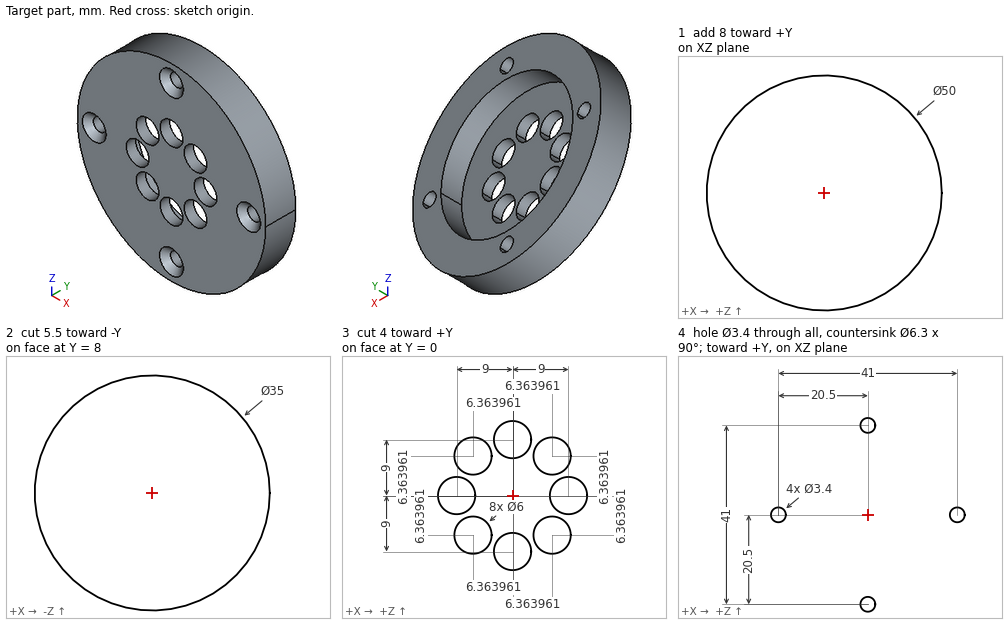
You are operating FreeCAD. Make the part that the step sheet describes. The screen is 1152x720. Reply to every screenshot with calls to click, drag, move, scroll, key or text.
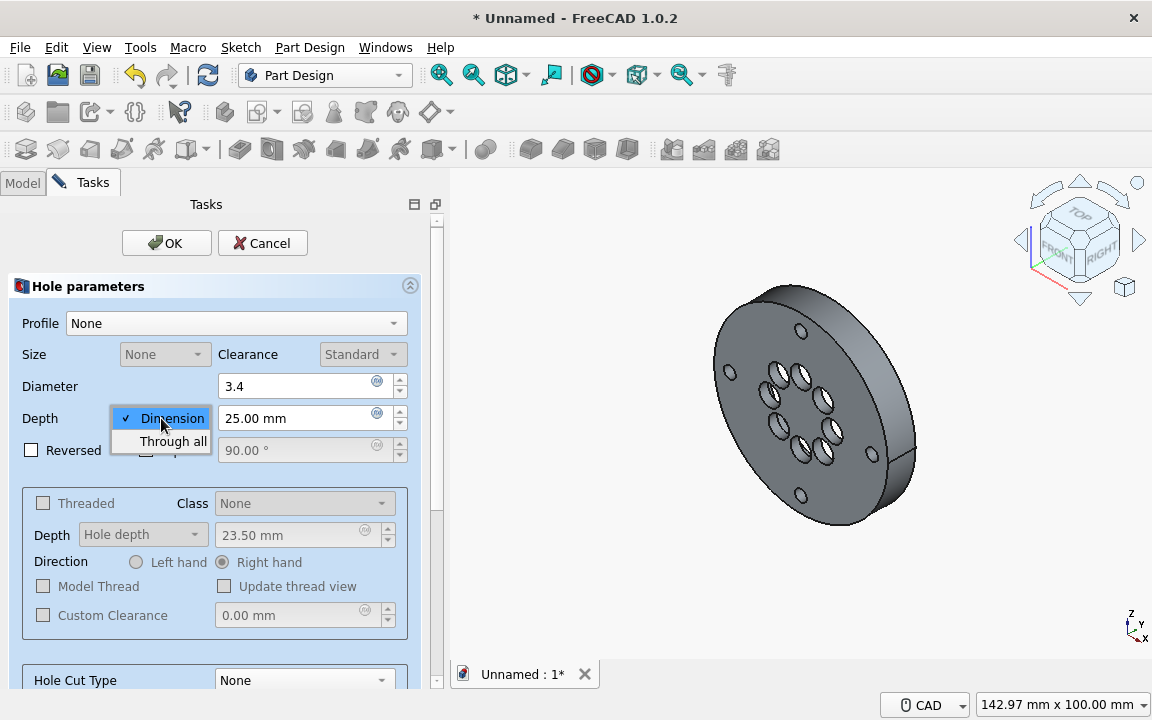
click(160, 442)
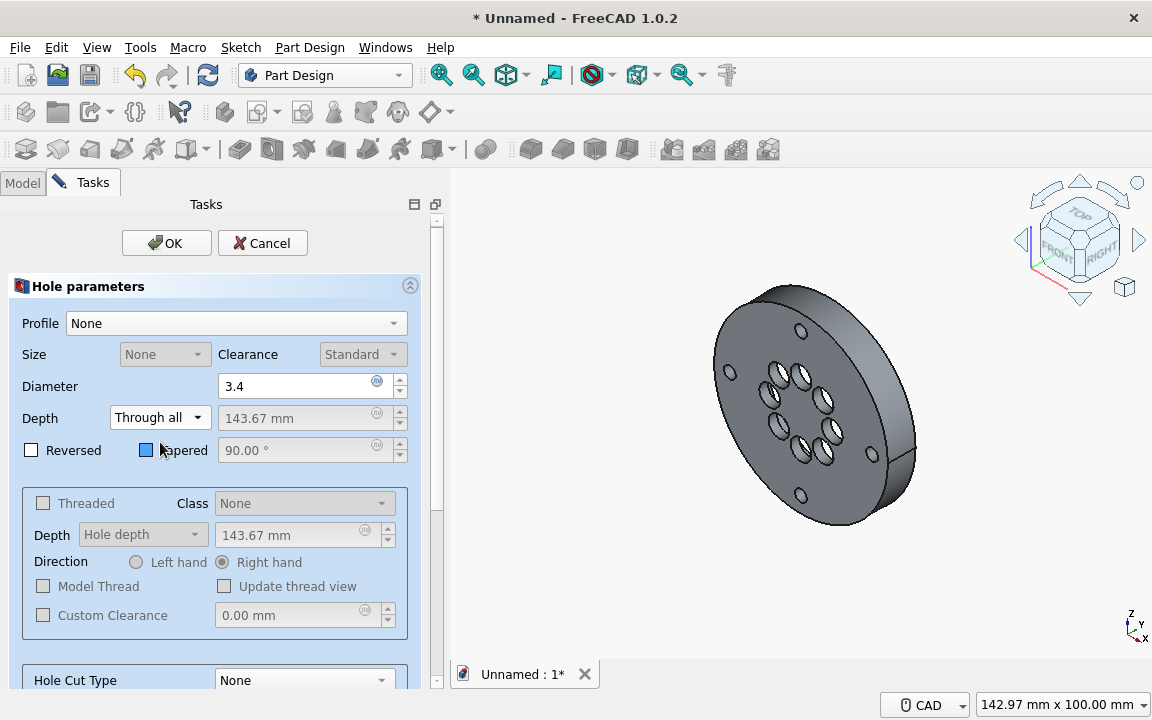
scroll(437, 451, down, 2)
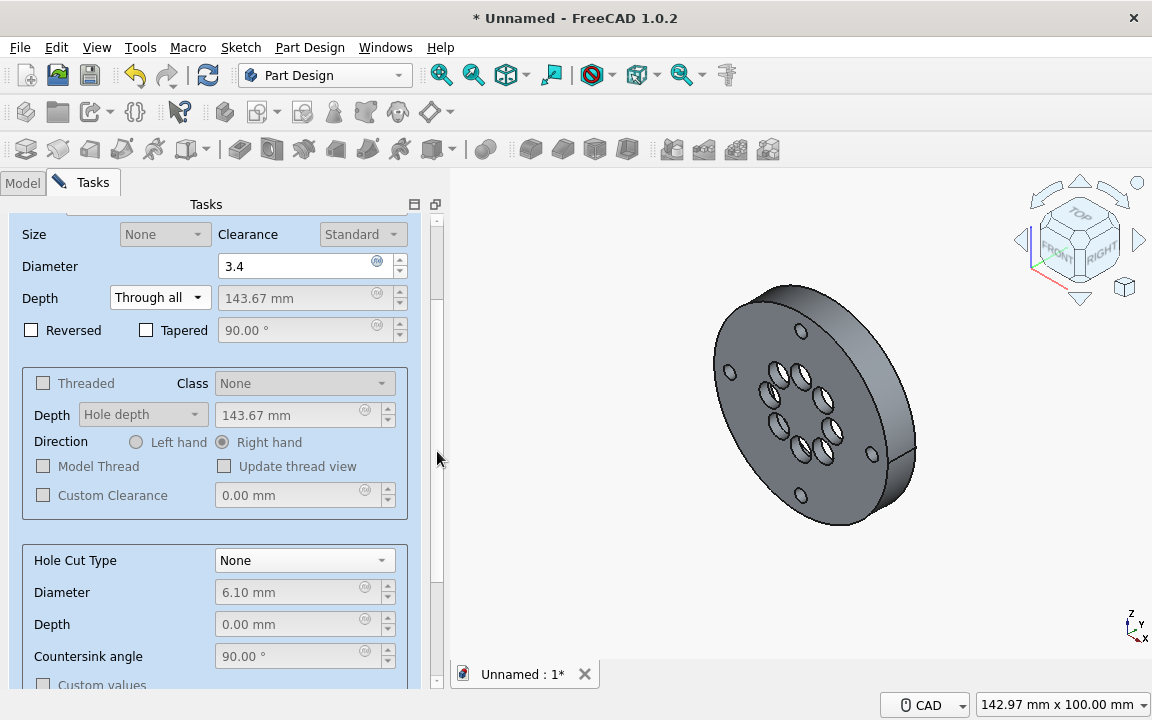
click(306, 560)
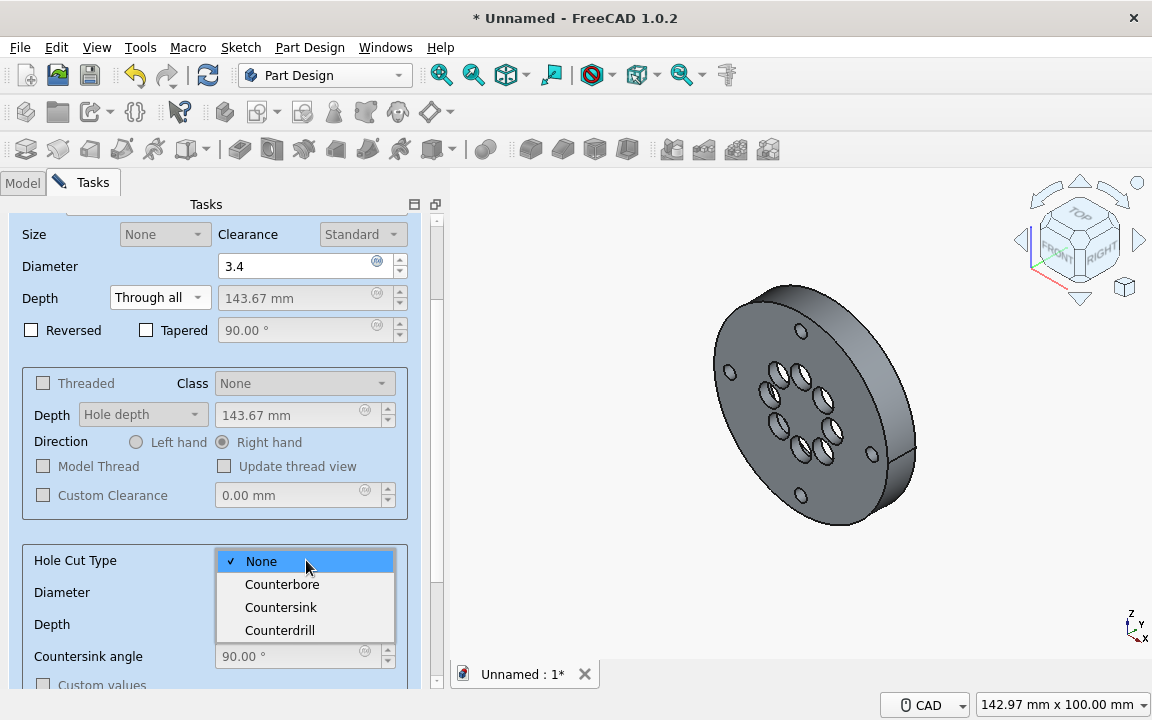
click(304, 608)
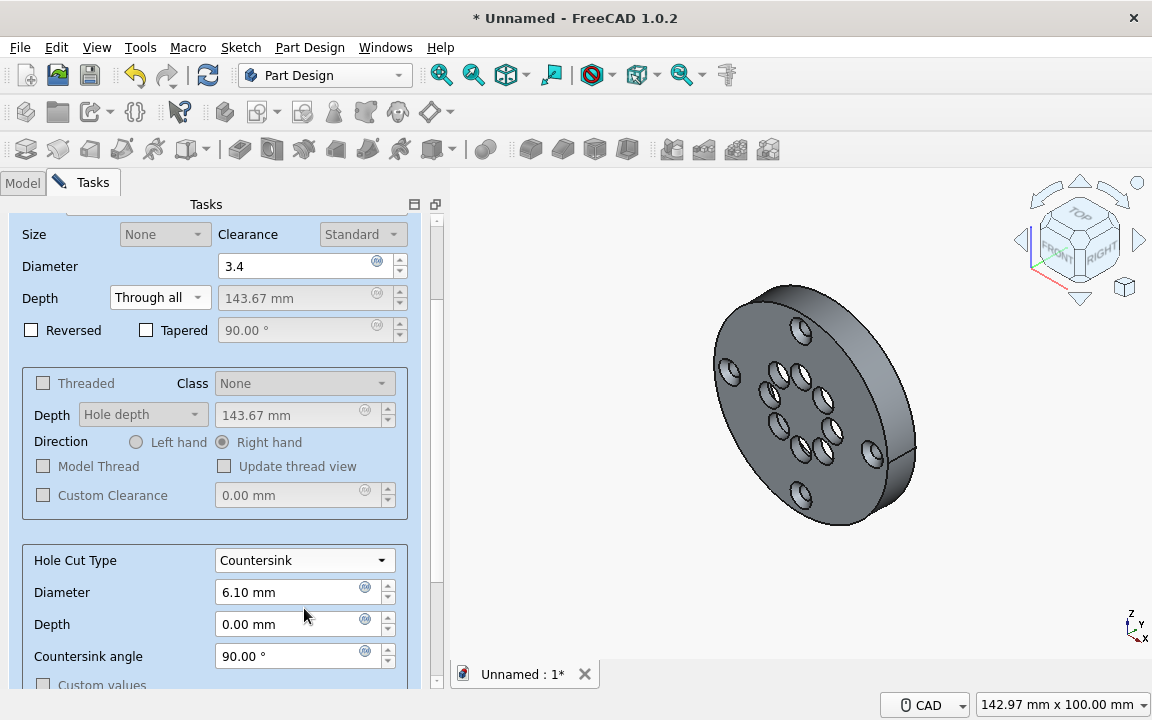
triple_click(298, 592)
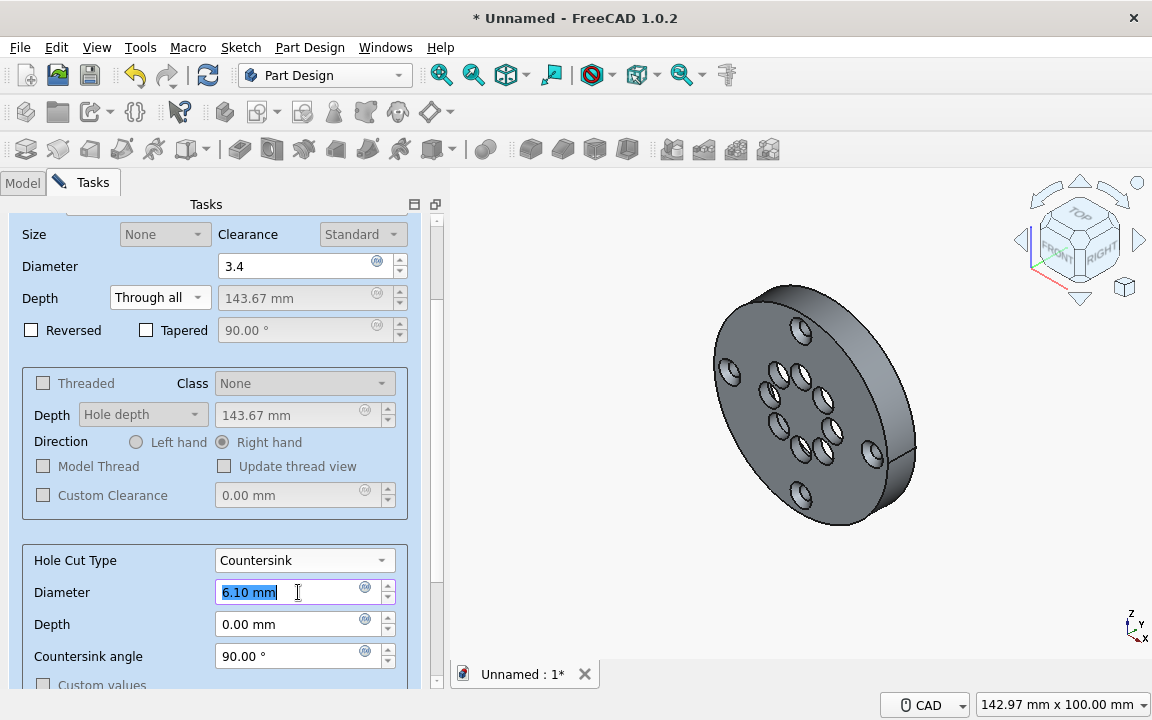
text(6.3)
key(Tab)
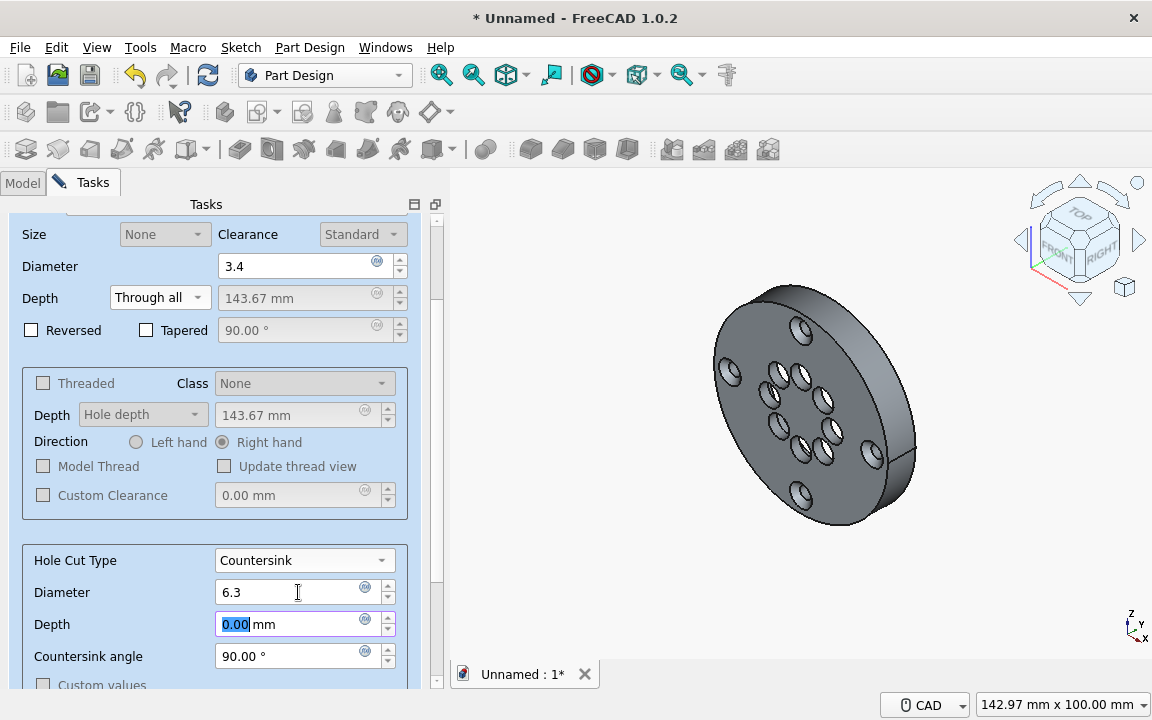
scroll(437, 451, up, 3)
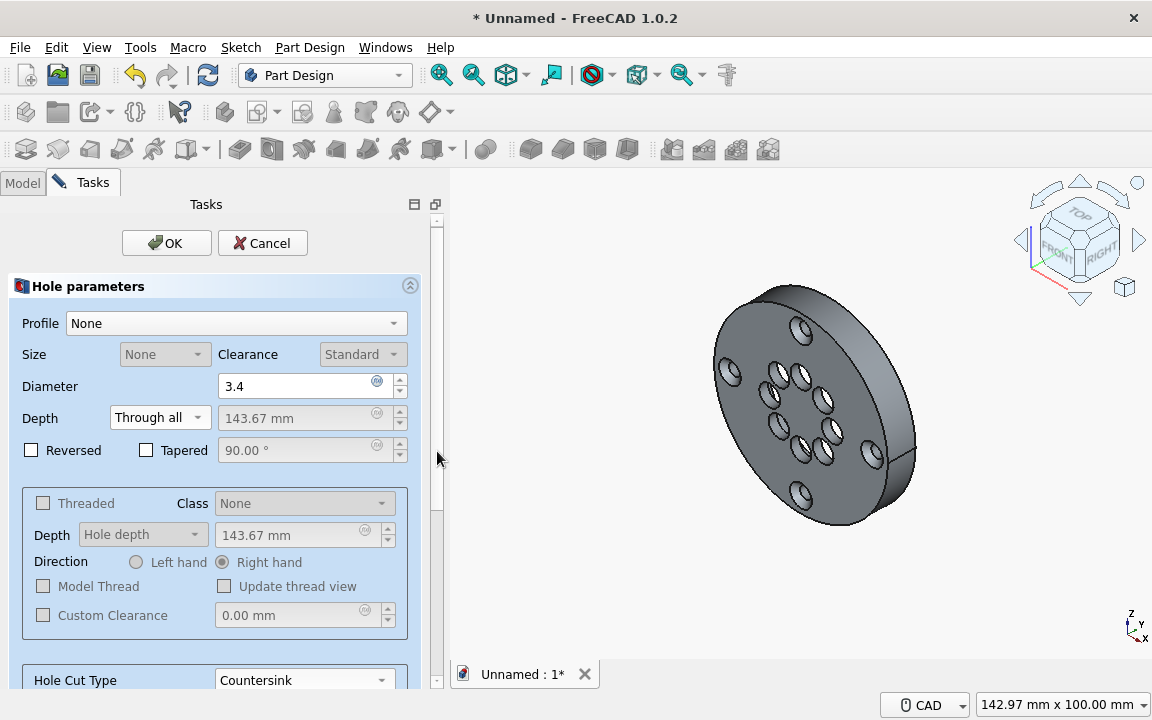
click(167, 243)